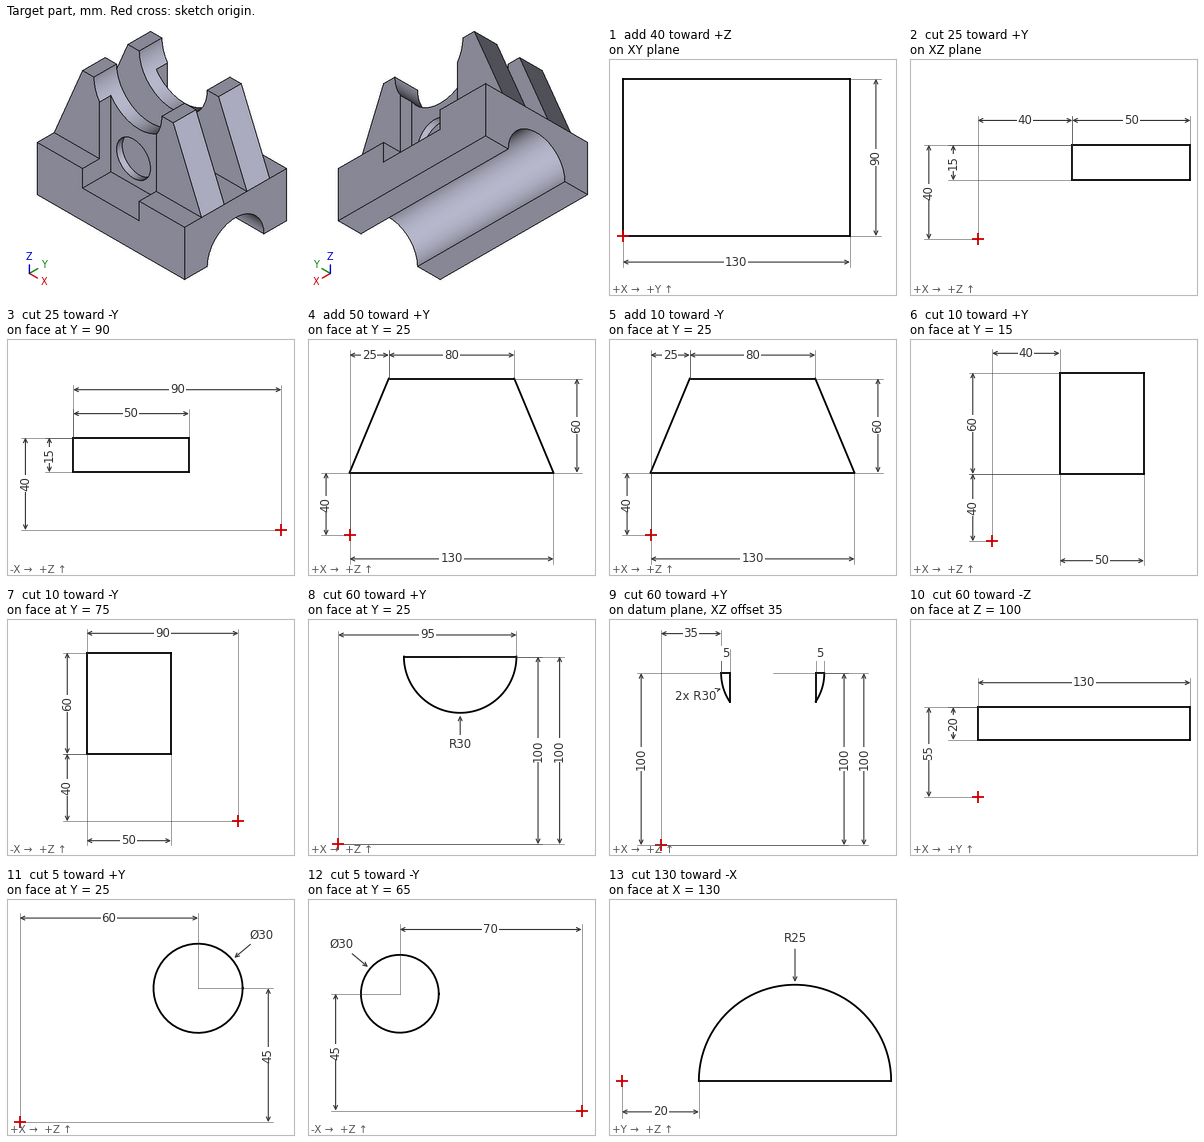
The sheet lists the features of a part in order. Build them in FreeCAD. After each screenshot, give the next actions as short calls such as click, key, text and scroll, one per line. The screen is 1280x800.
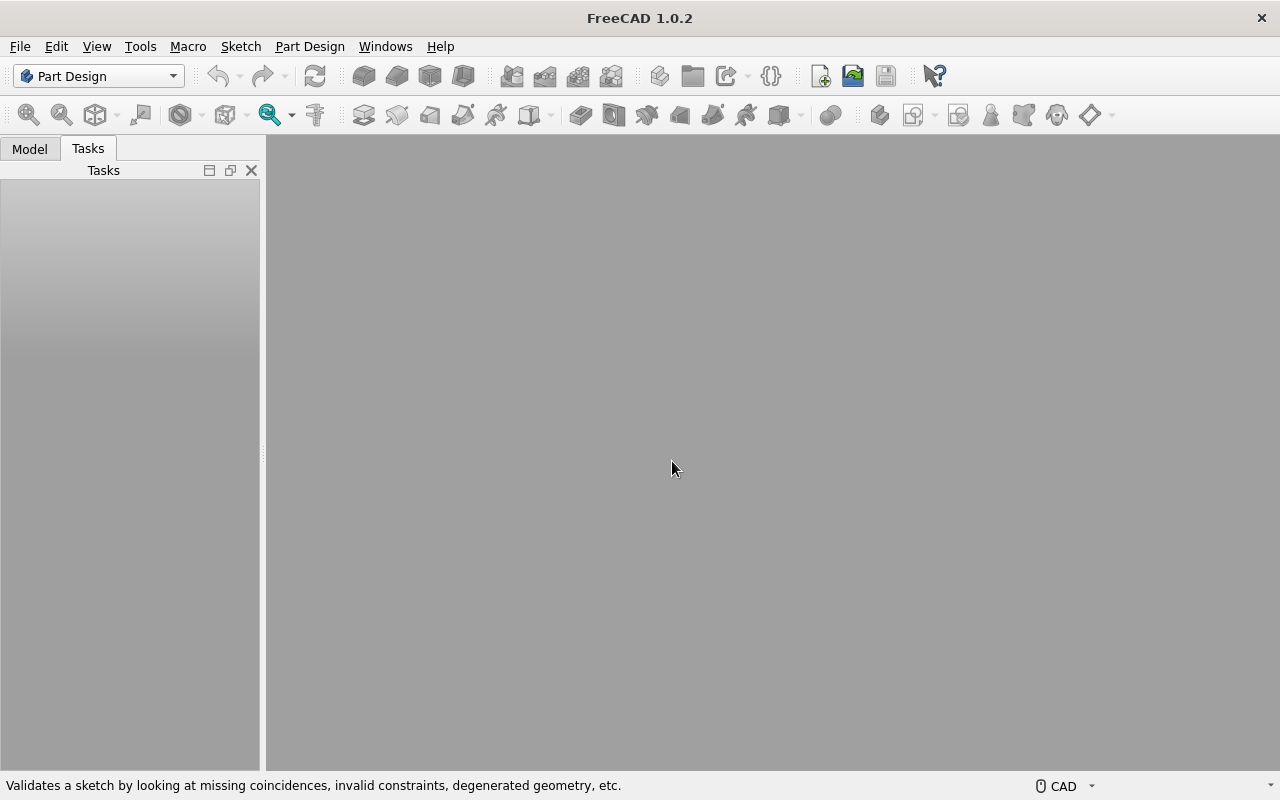
click(820, 76)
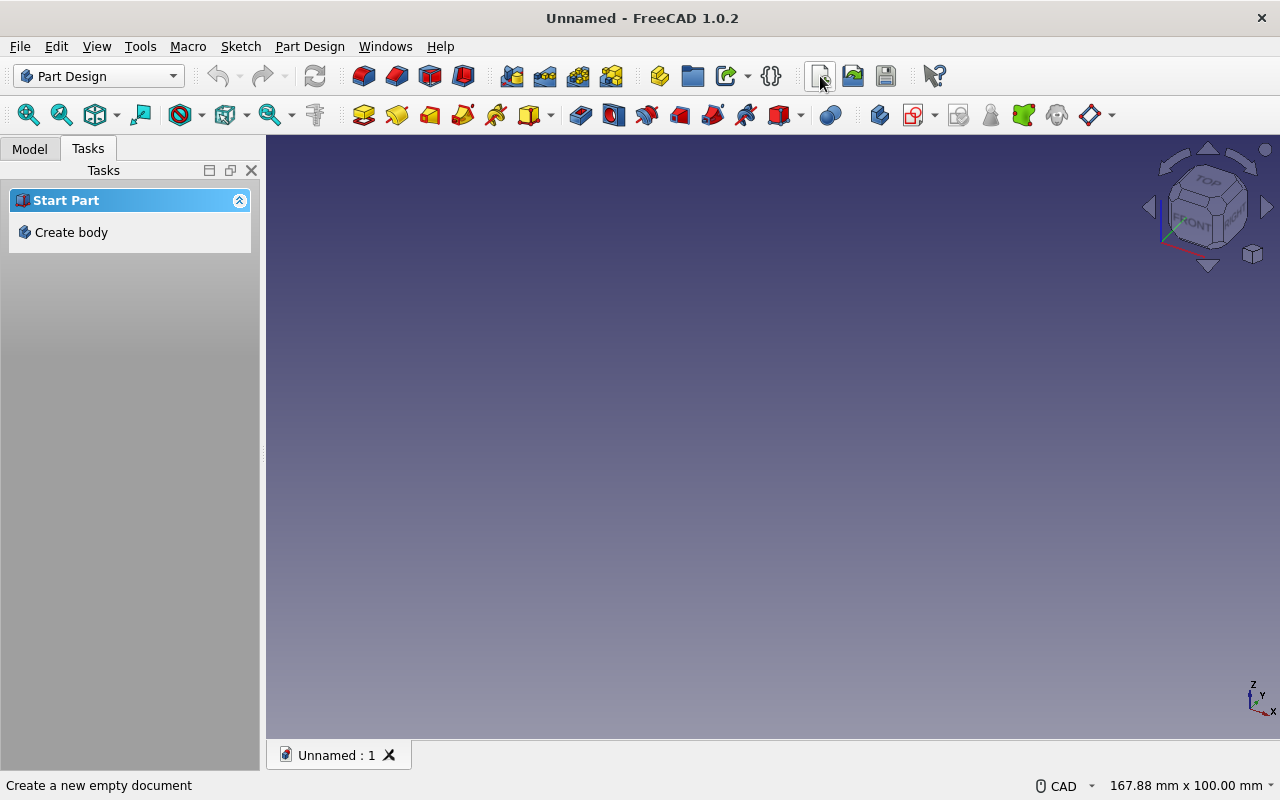
click(912, 116)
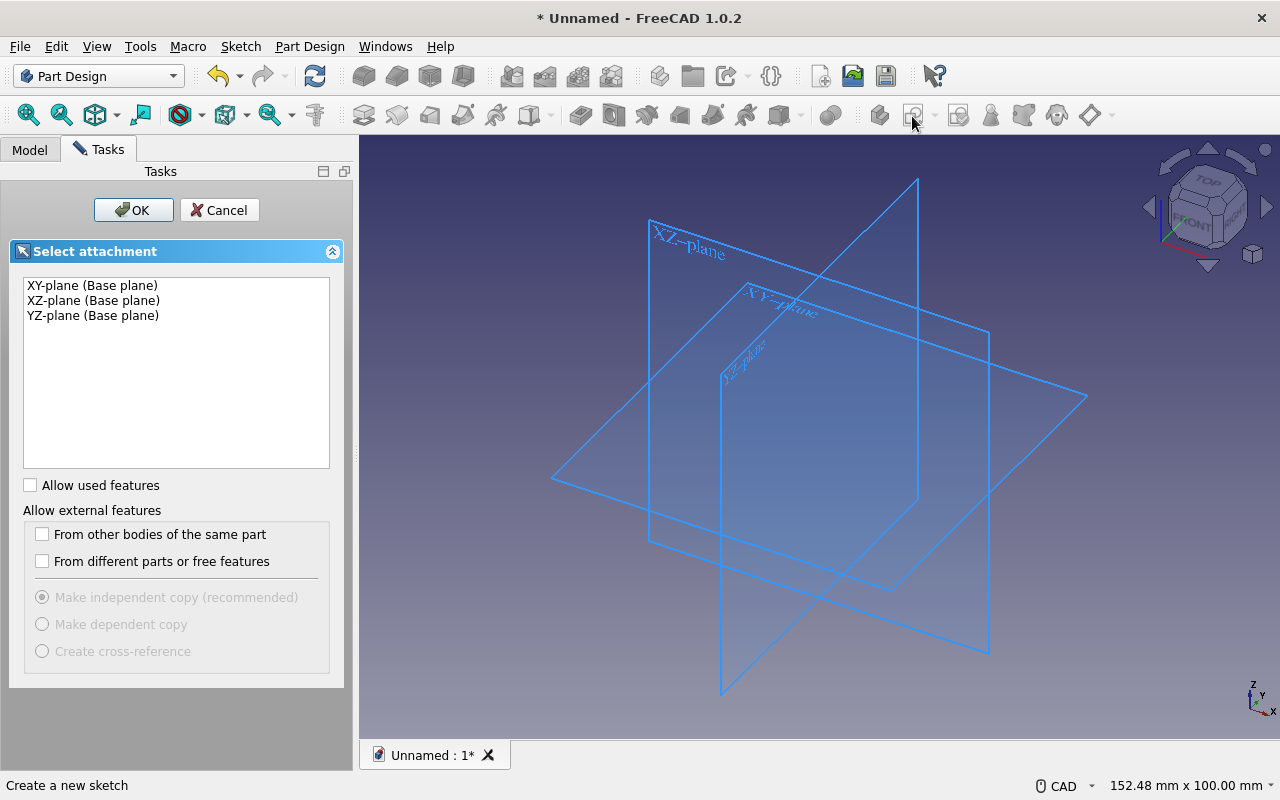
click(84, 286)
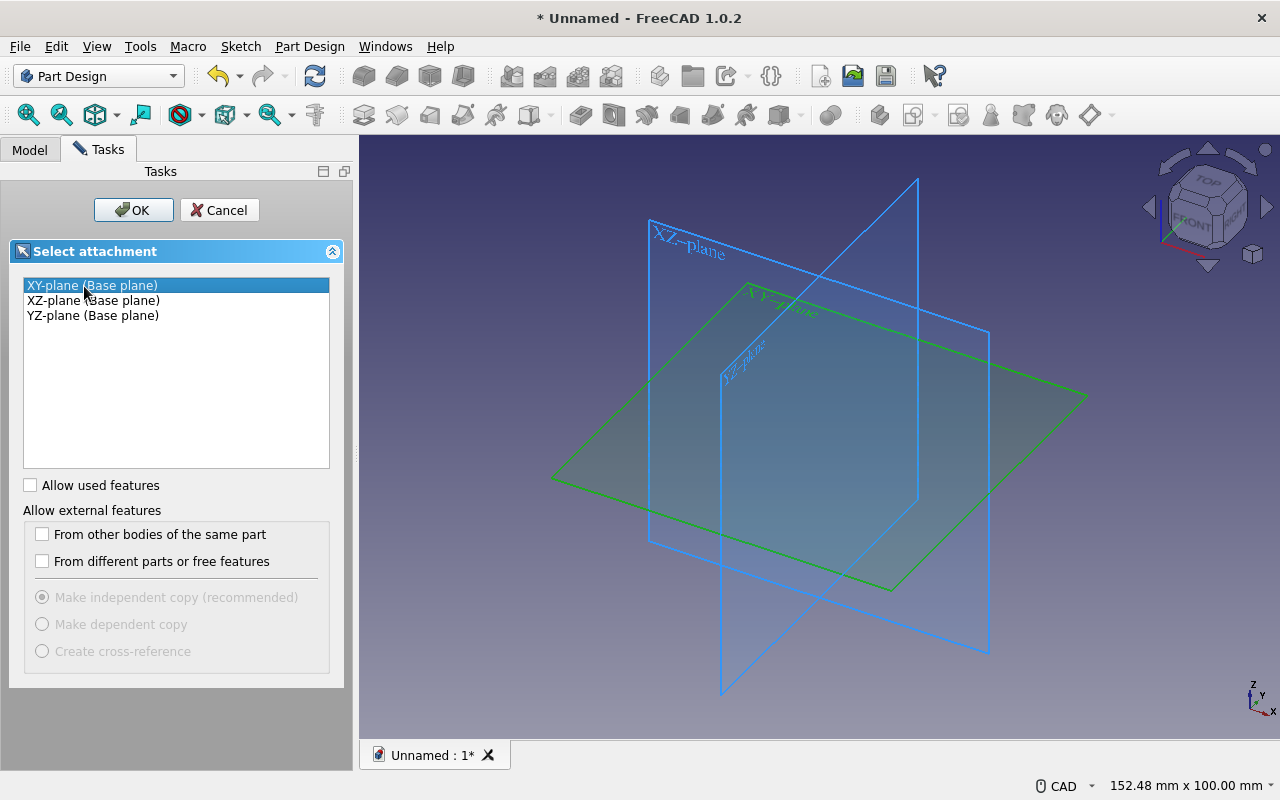
click(134, 210)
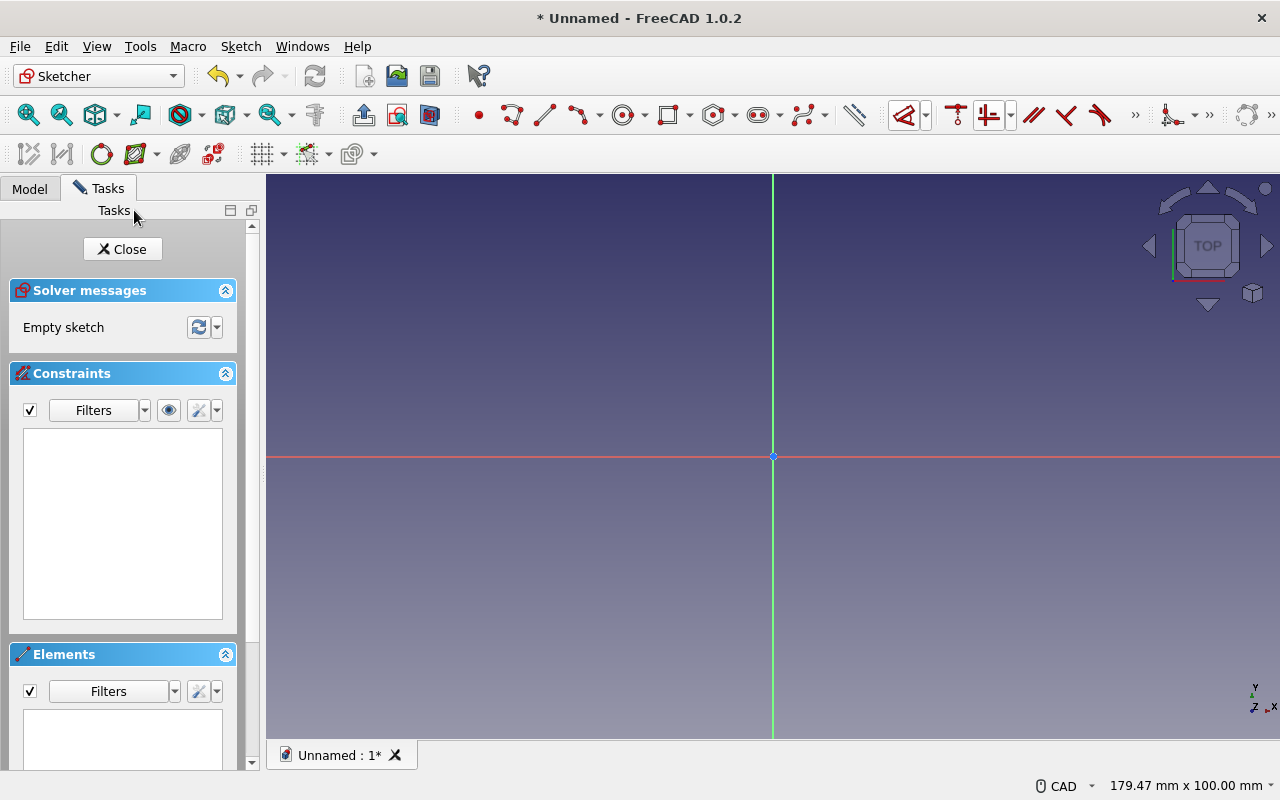
scroll(294, 711, down, 3)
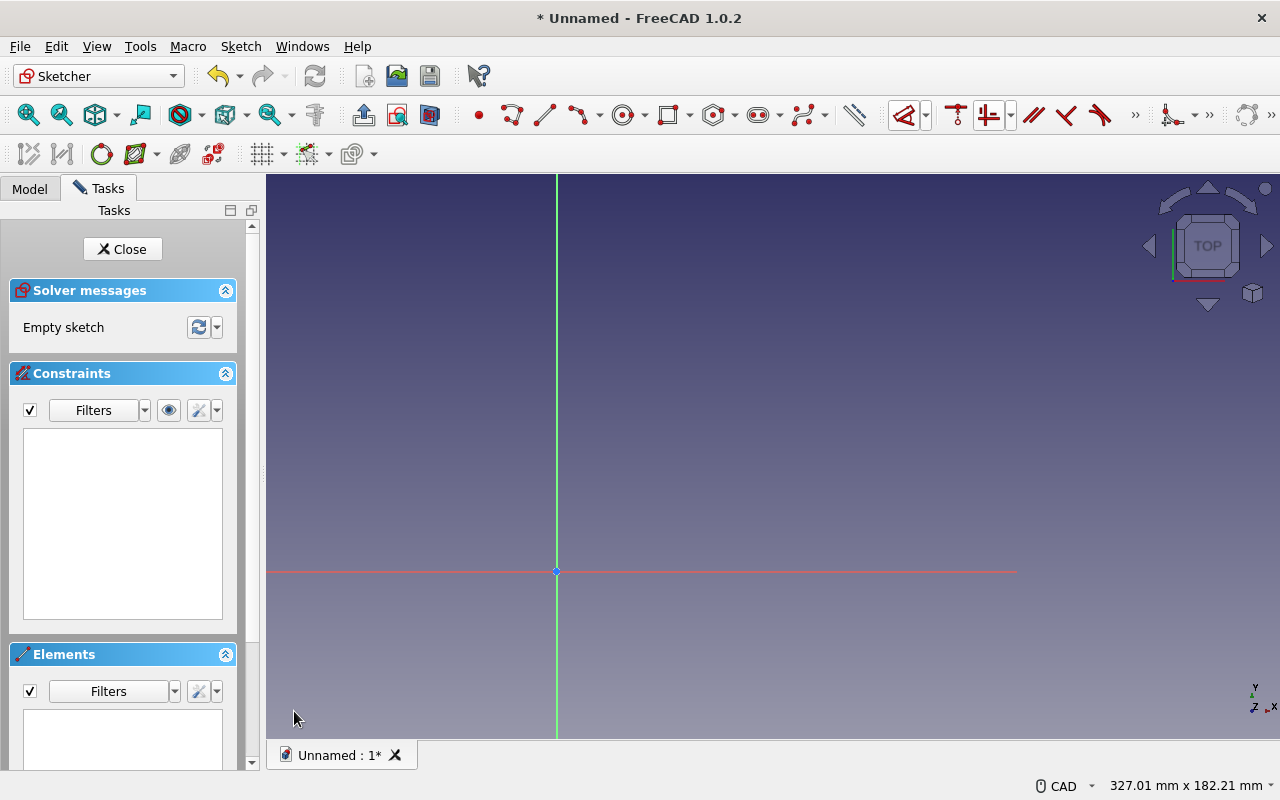
click(668, 116)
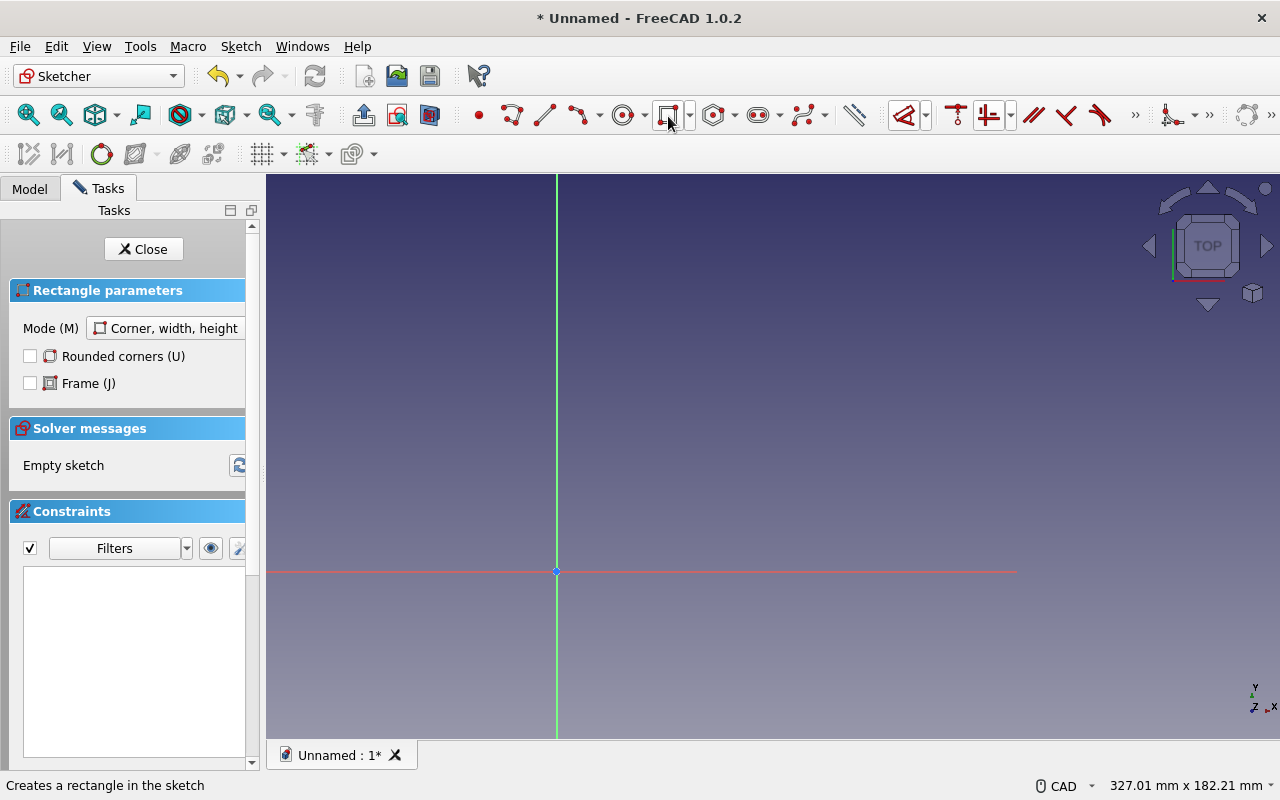
click(557, 572)
click(960, 293)
key(Escape)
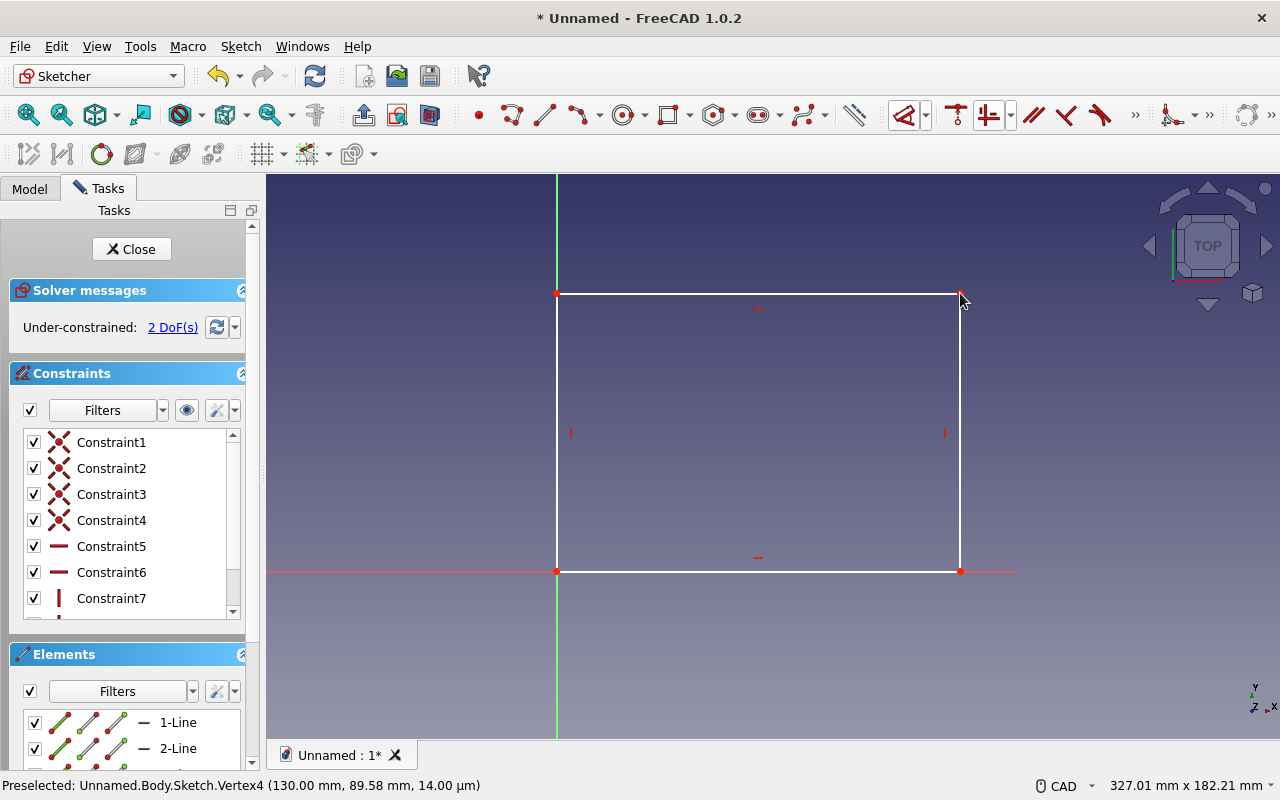
key(d)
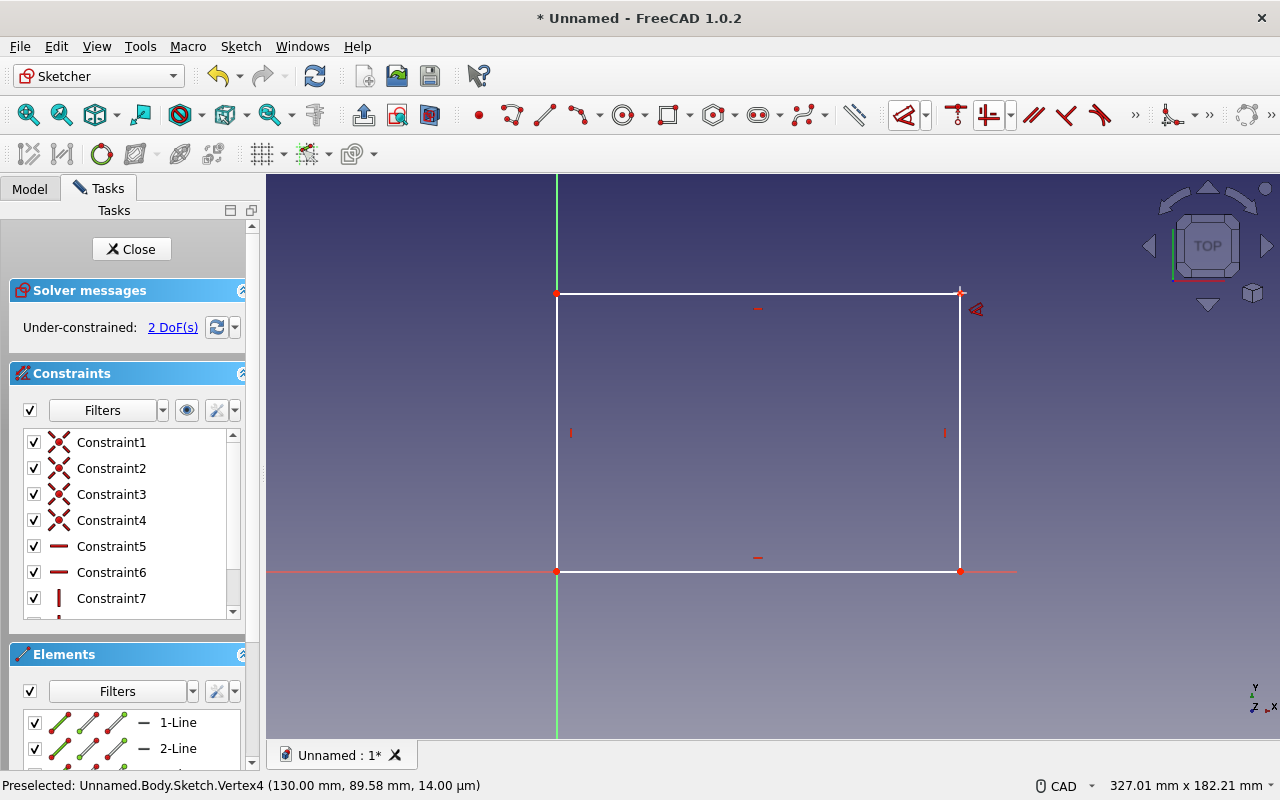
click(960, 488)
click(994, 433)